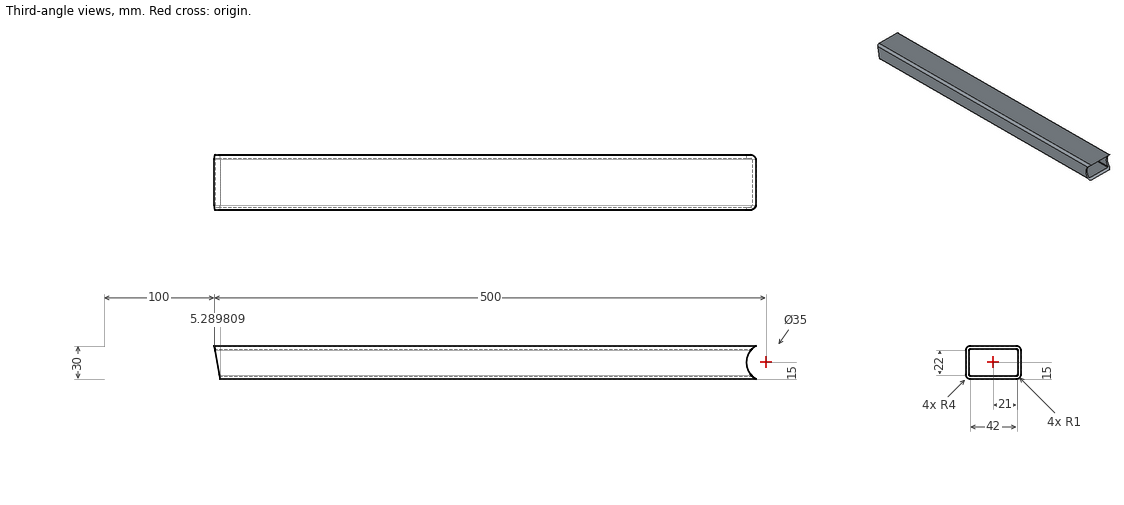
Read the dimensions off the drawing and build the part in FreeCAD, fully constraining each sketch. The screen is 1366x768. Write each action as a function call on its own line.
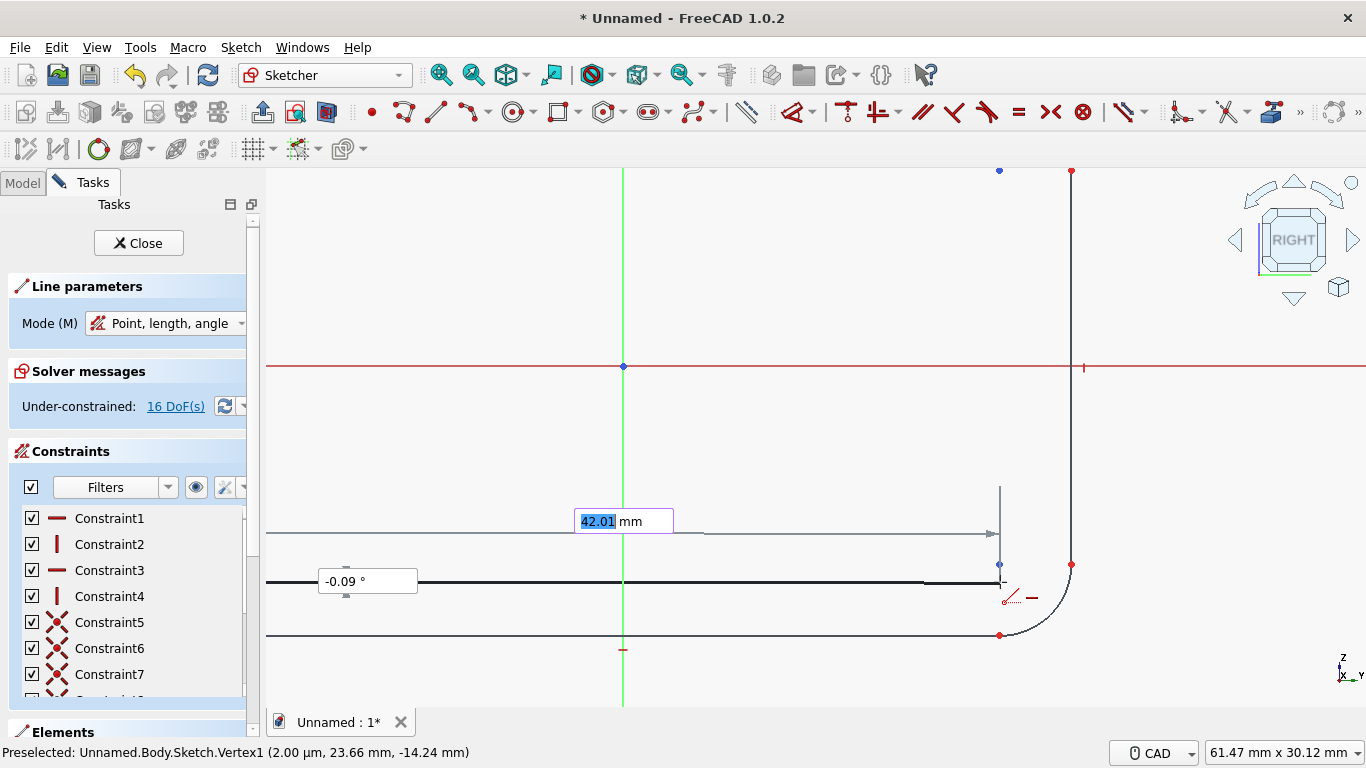
click(999, 581)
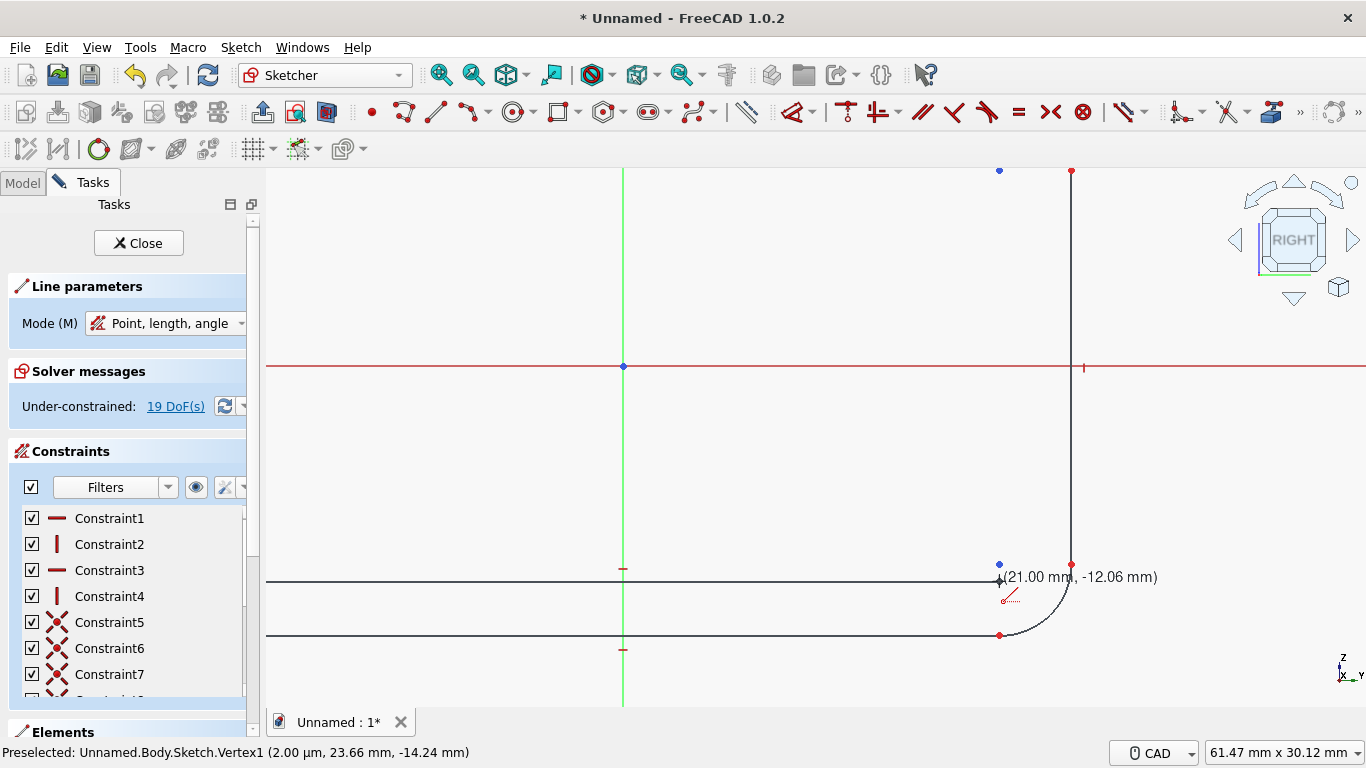
click(1017, 563)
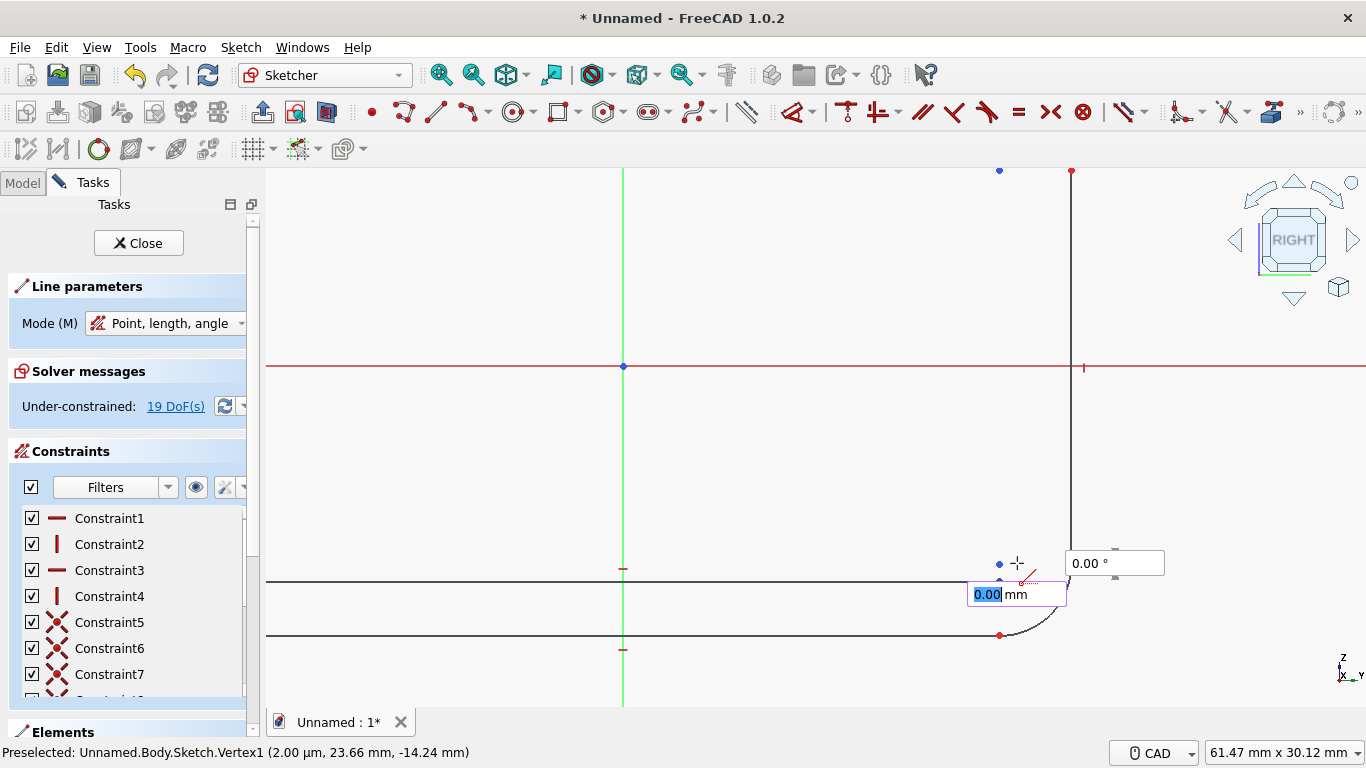
scroll(1000, 582, down, 2)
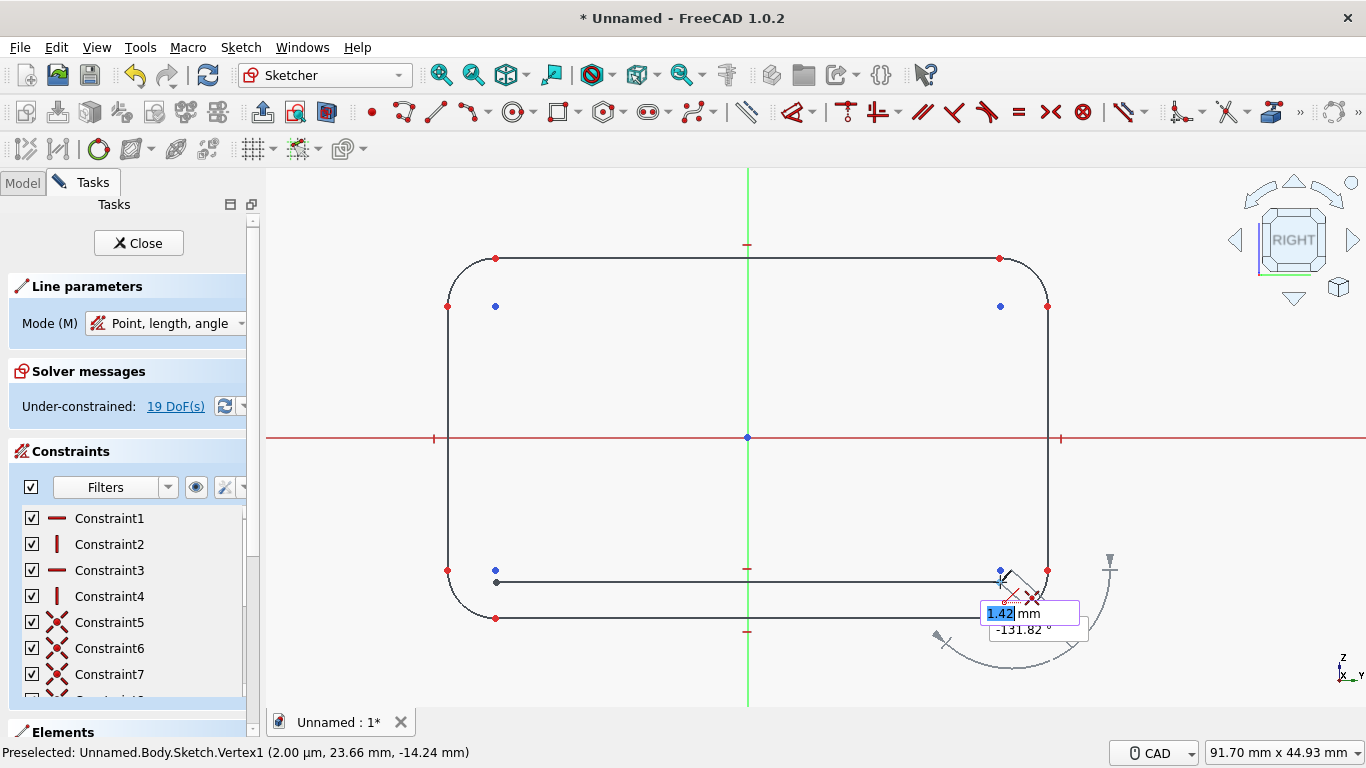
scroll(1012, 306, up, 2)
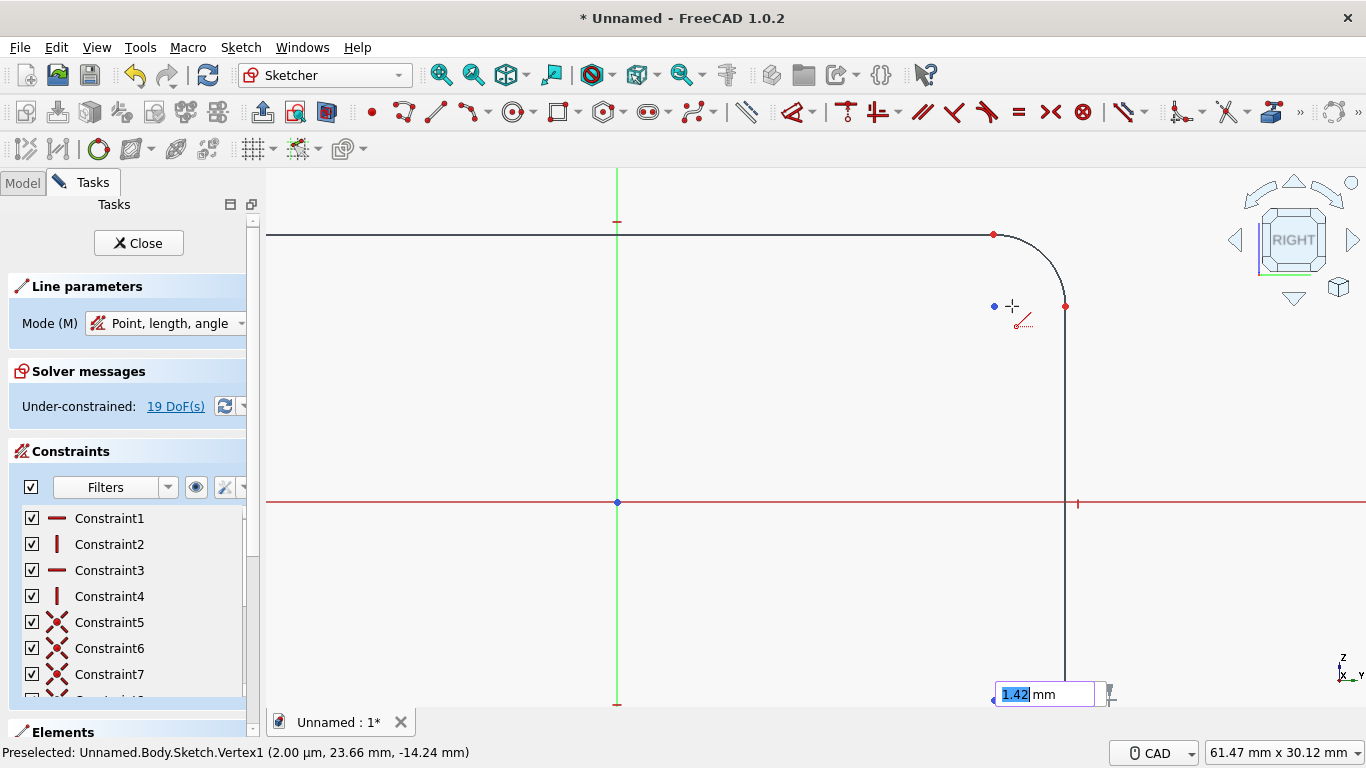
click(1011, 305)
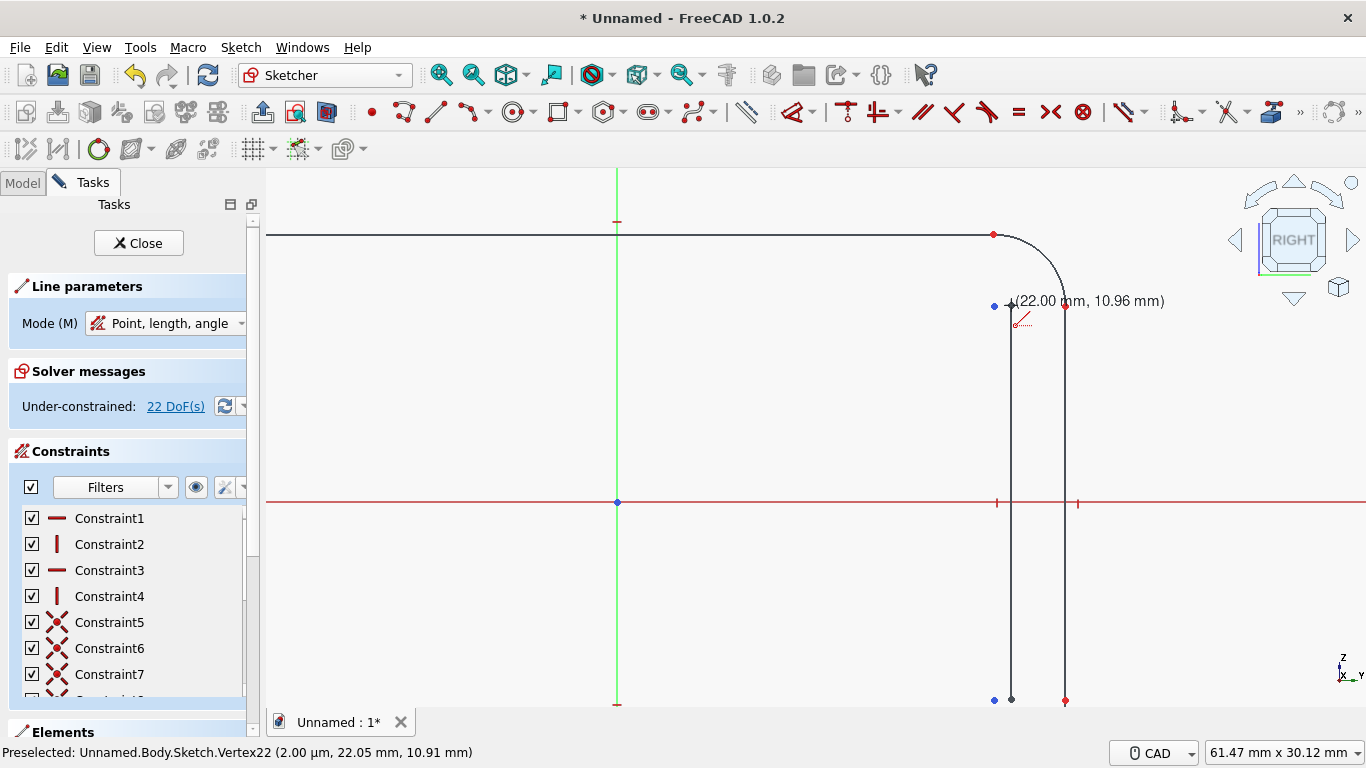
click(993, 287)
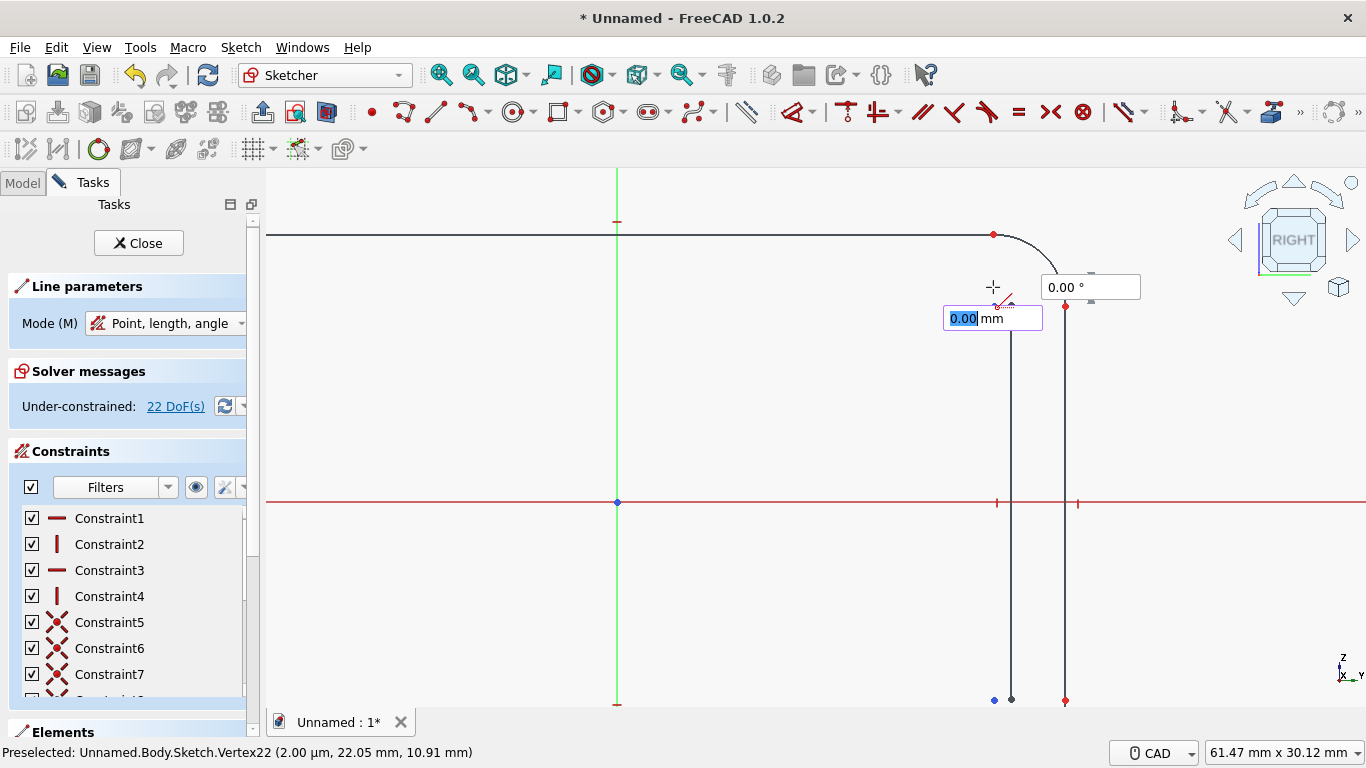
scroll(1012, 306, down, 2)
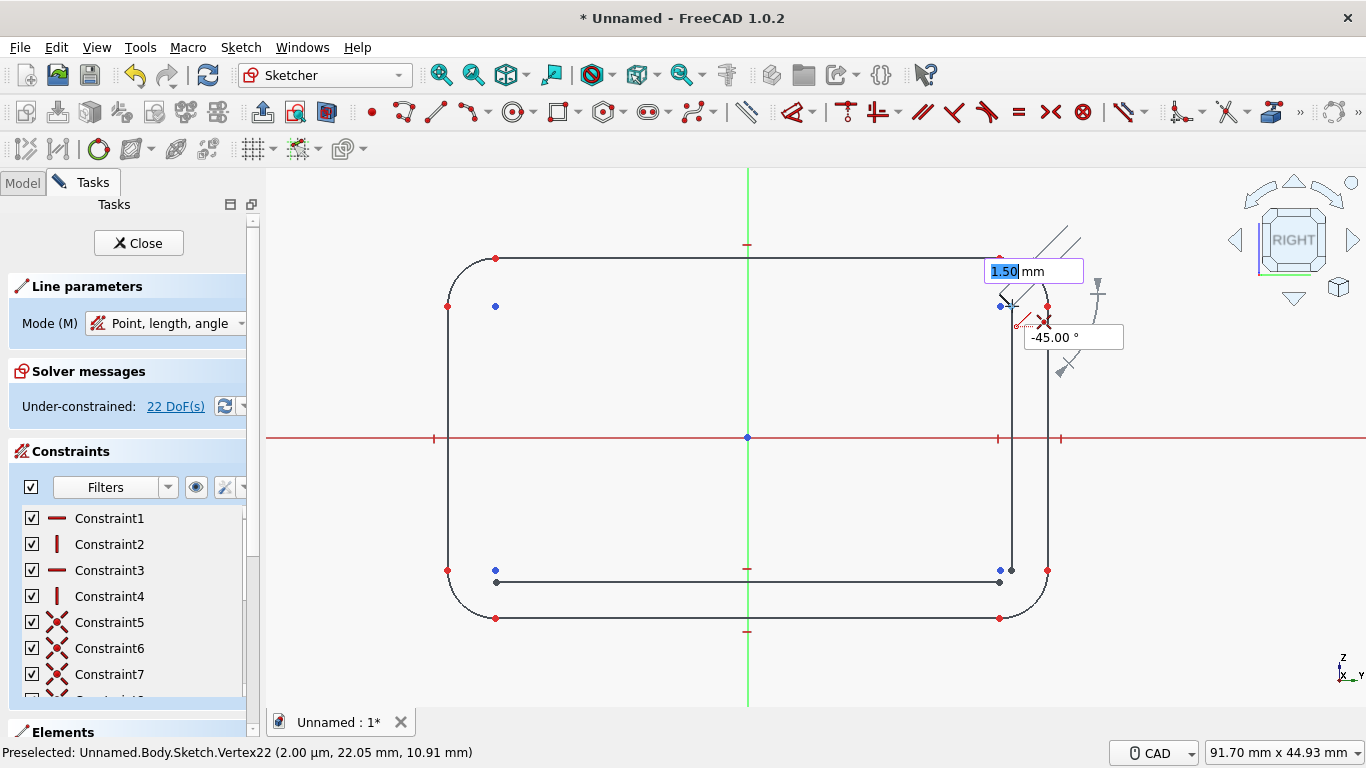
scroll(496, 294, up, 2)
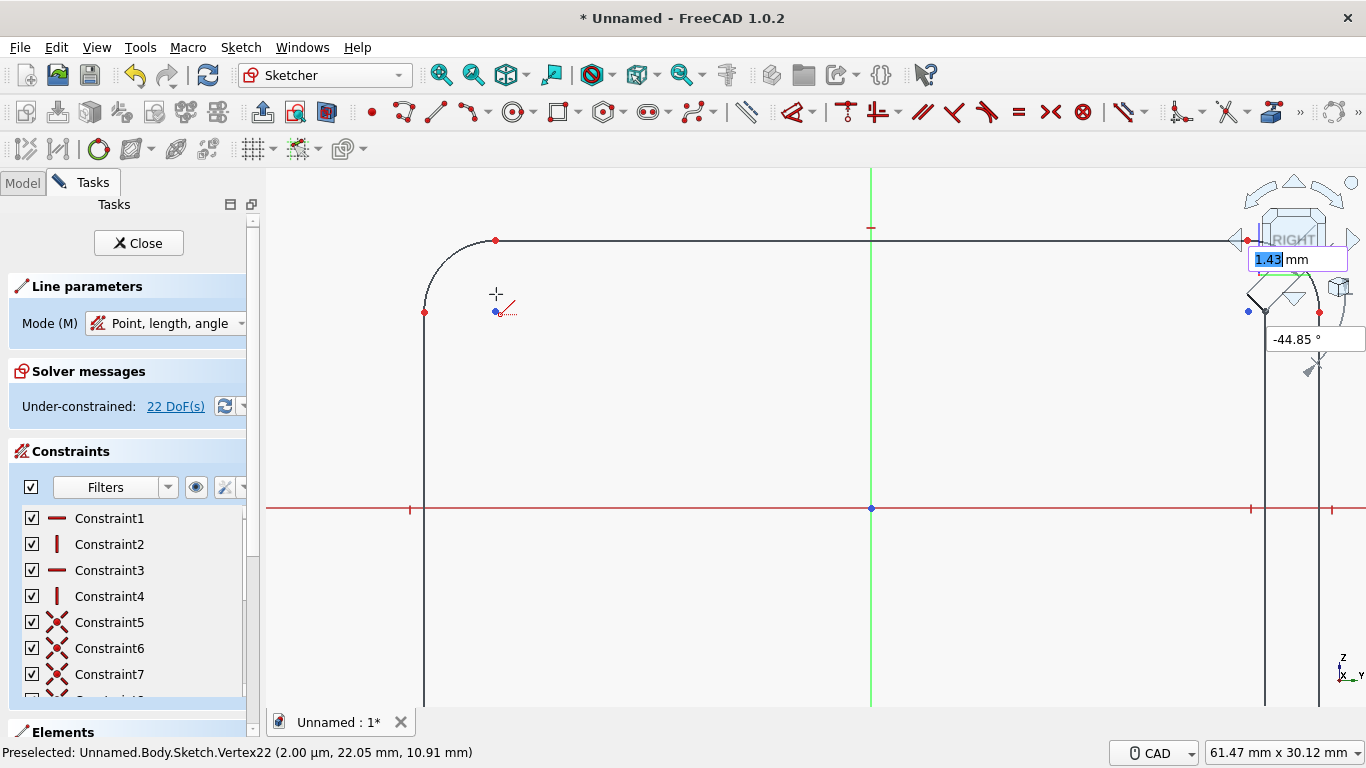
click(496, 293)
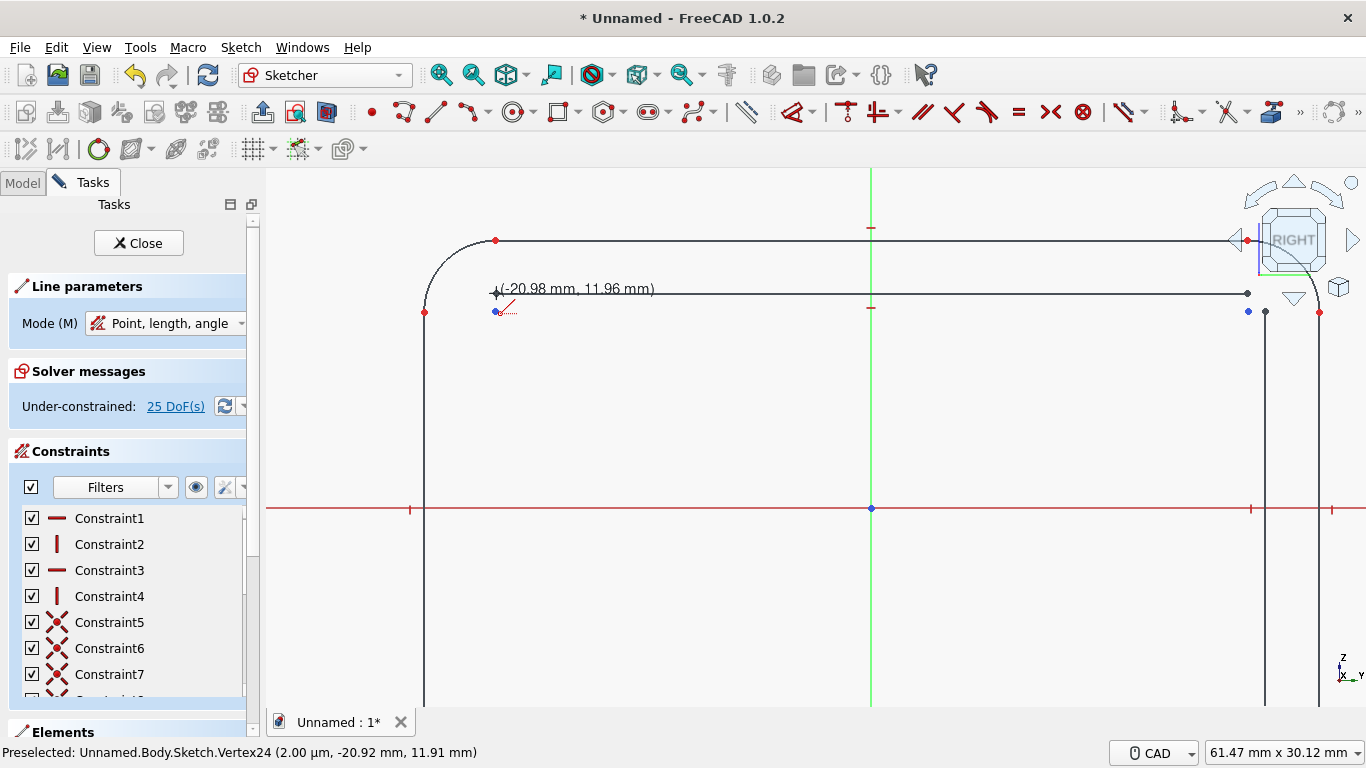
click(478, 311)